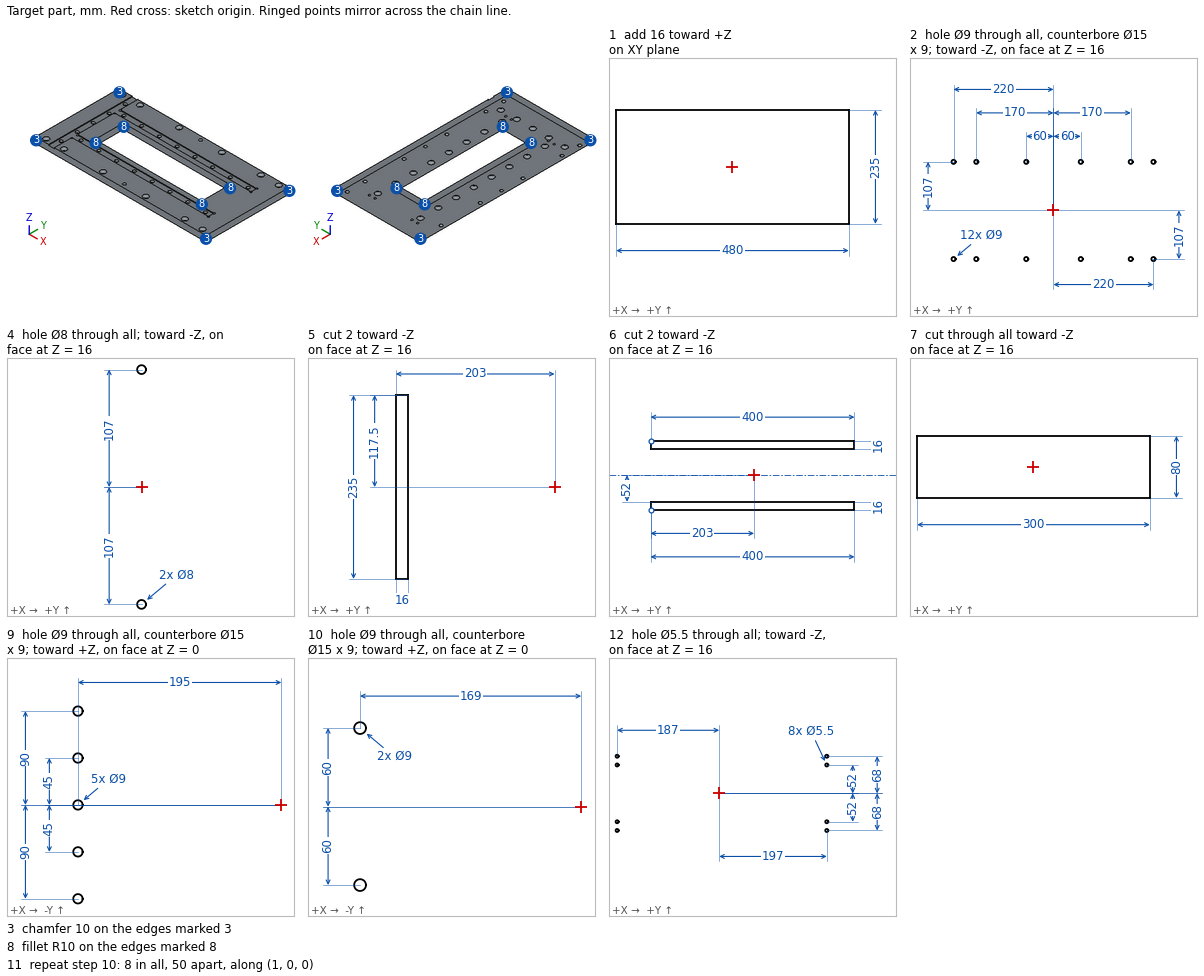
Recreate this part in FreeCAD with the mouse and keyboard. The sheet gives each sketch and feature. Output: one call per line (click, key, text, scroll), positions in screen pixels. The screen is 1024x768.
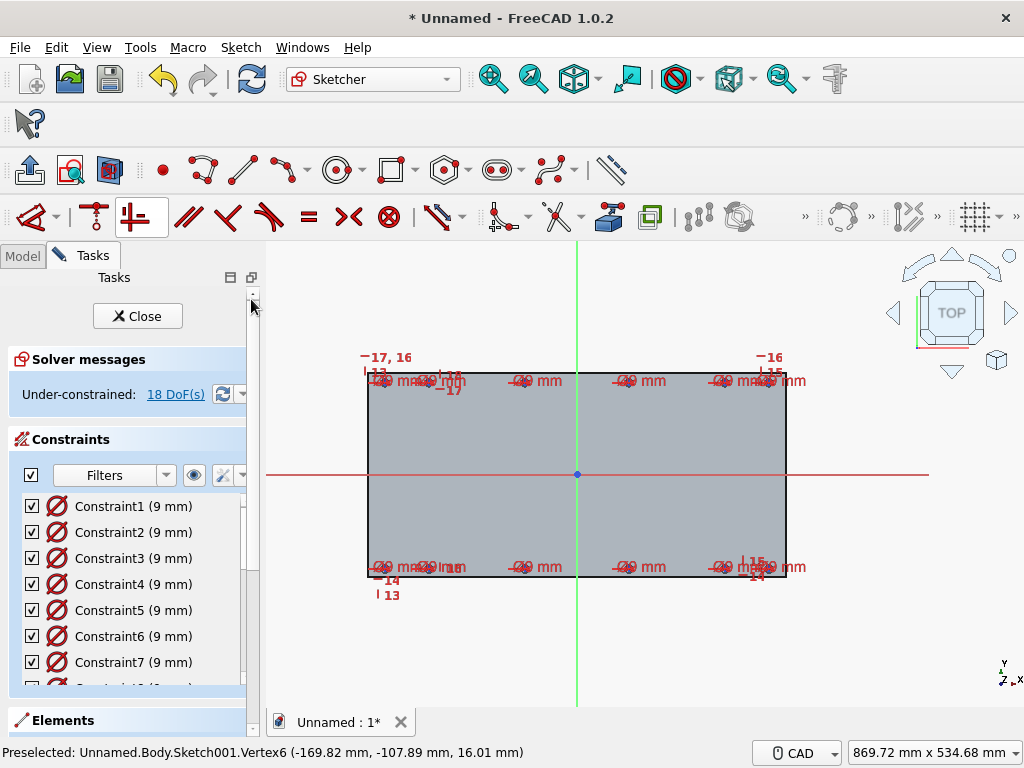
click(385, 569)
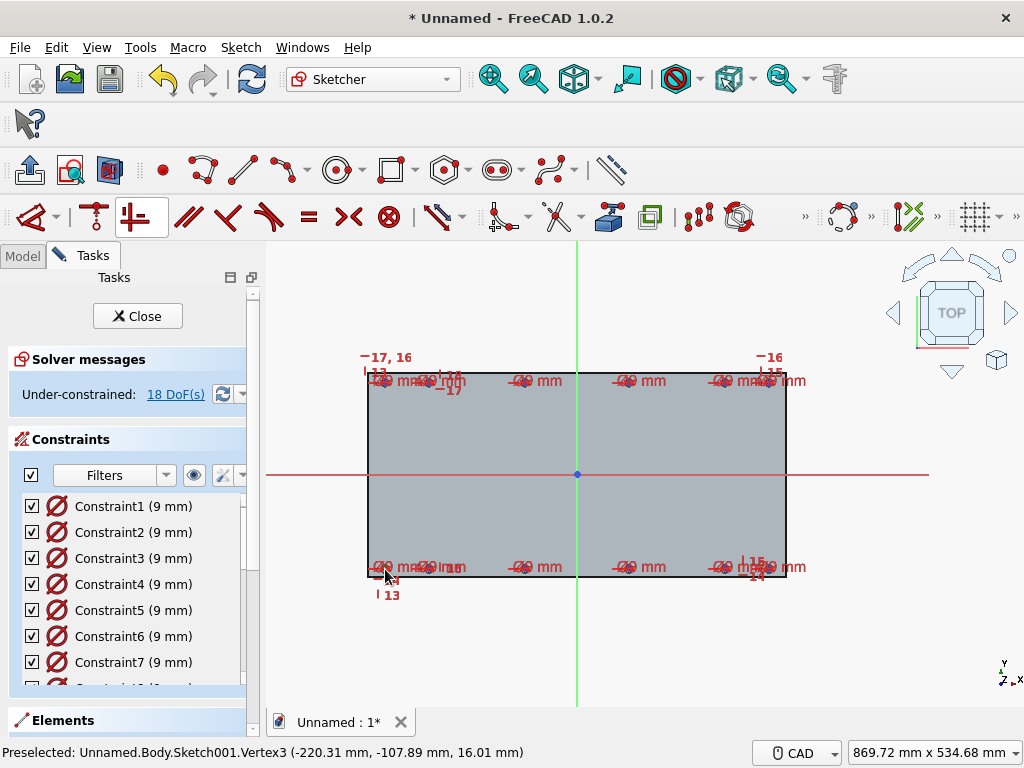
click(429, 569)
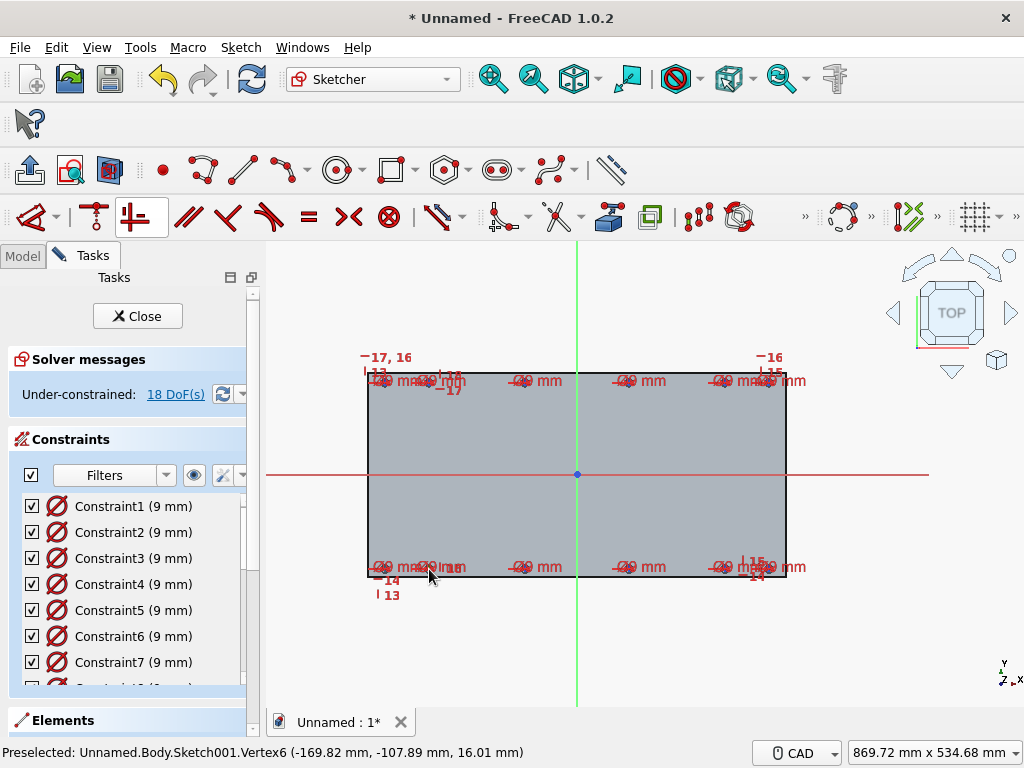
click(162, 218)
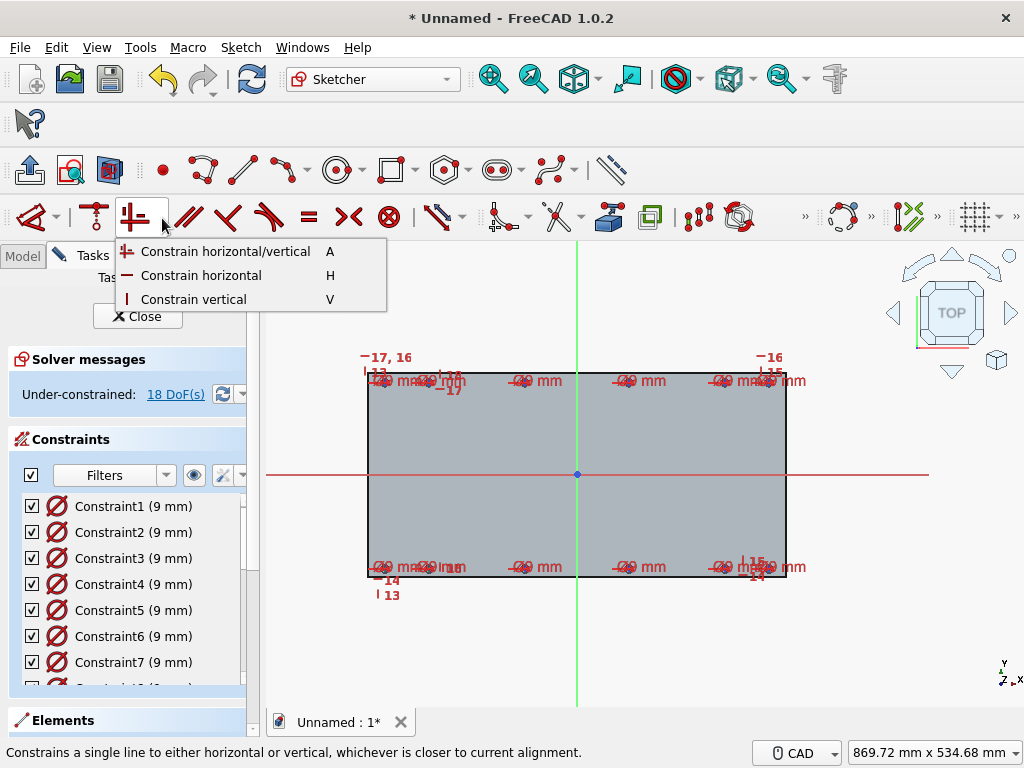
click(251, 275)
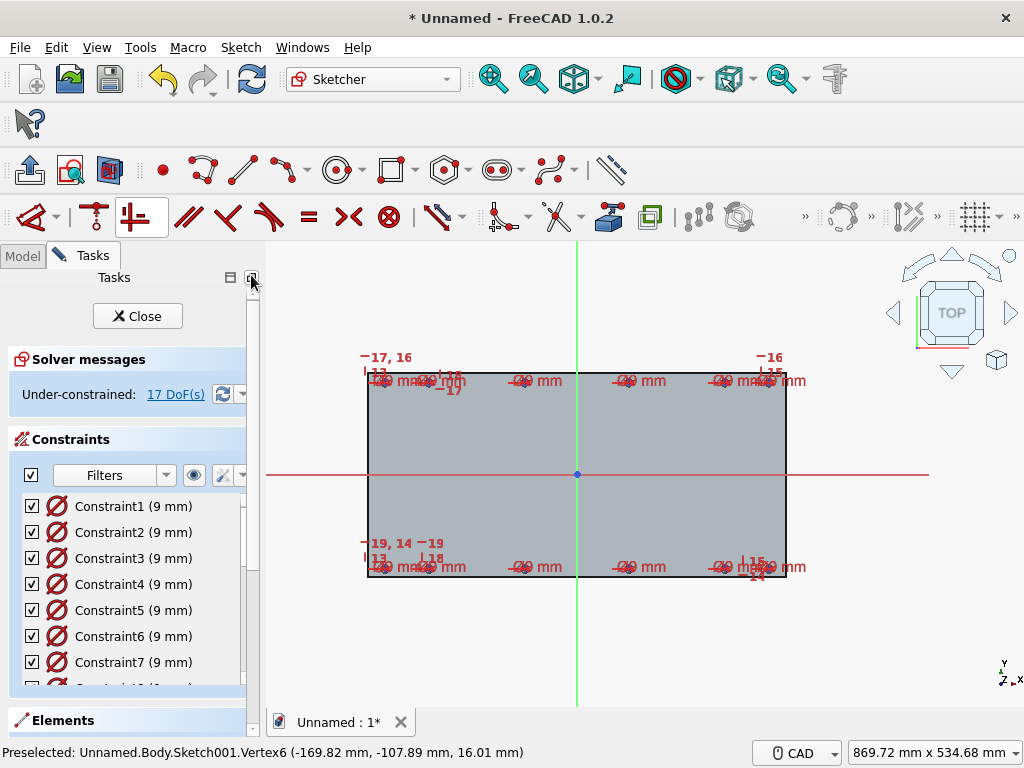
click(429, 383)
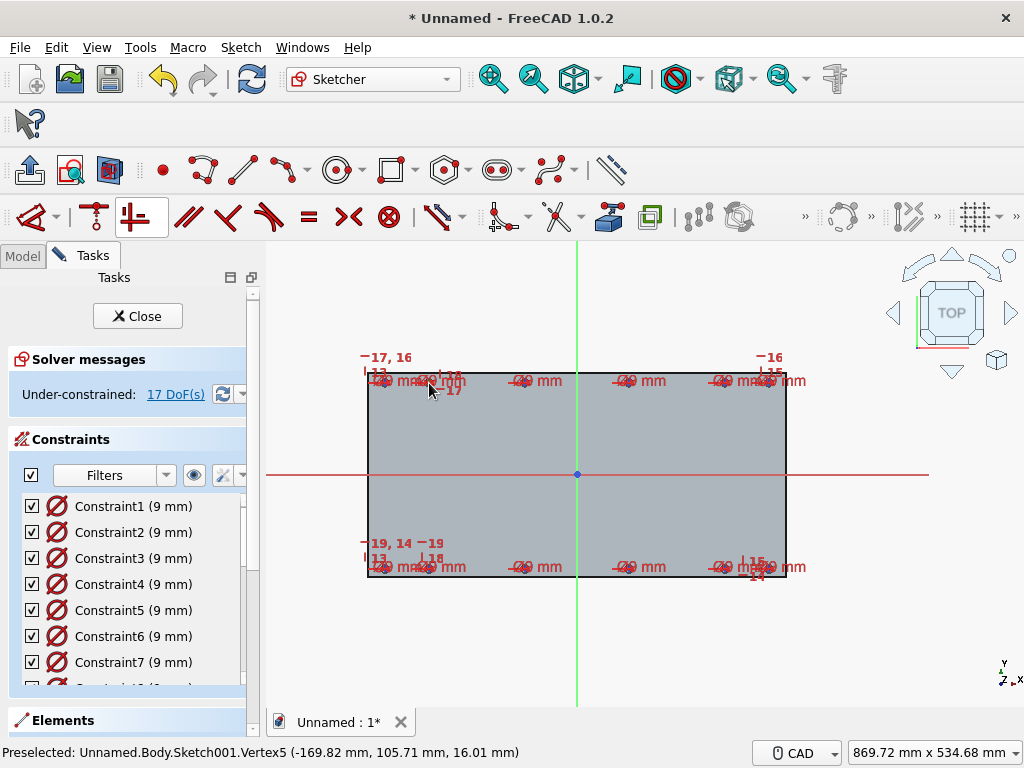
click(525, 383)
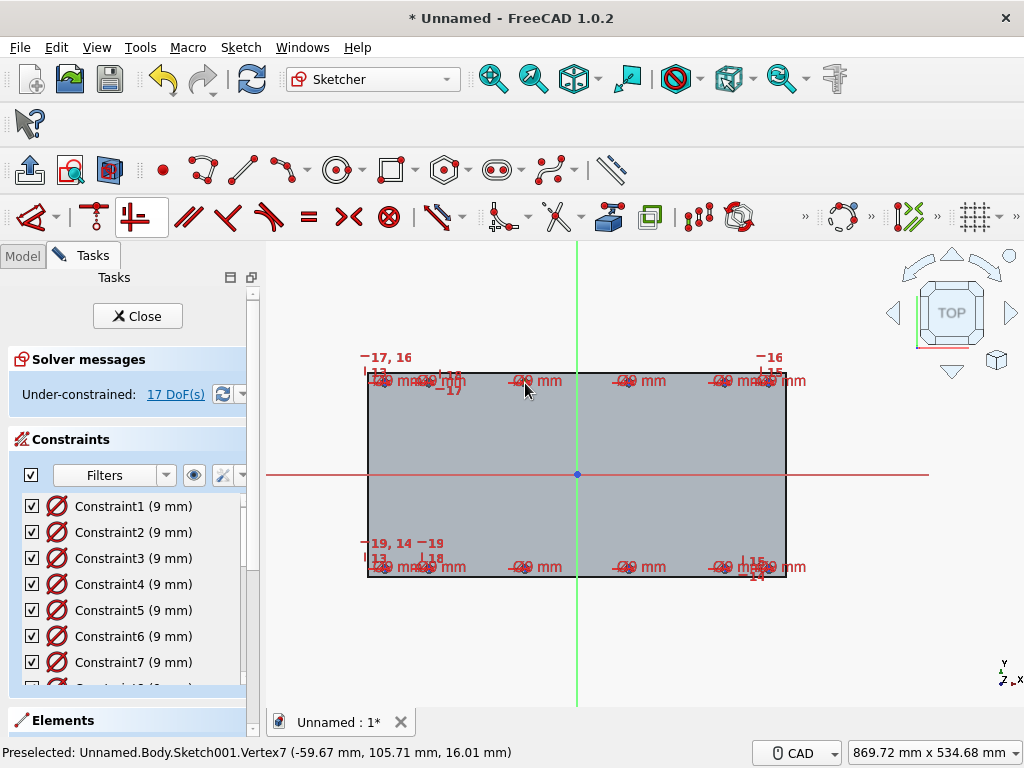
click(162, 218)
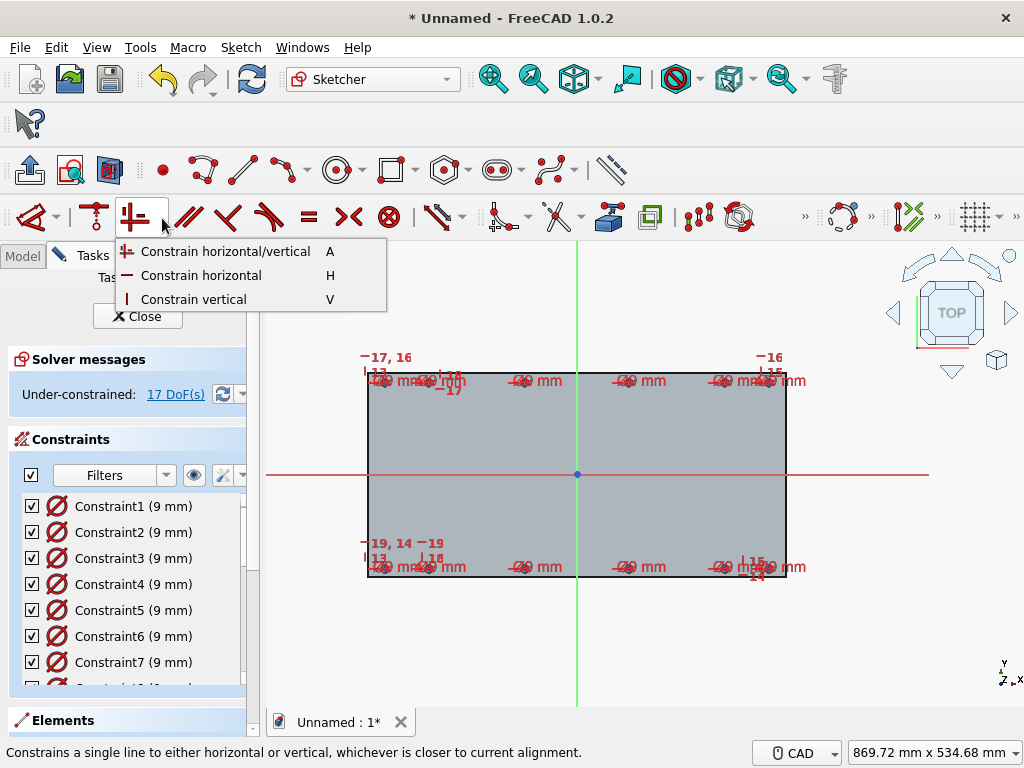
click(251, 275)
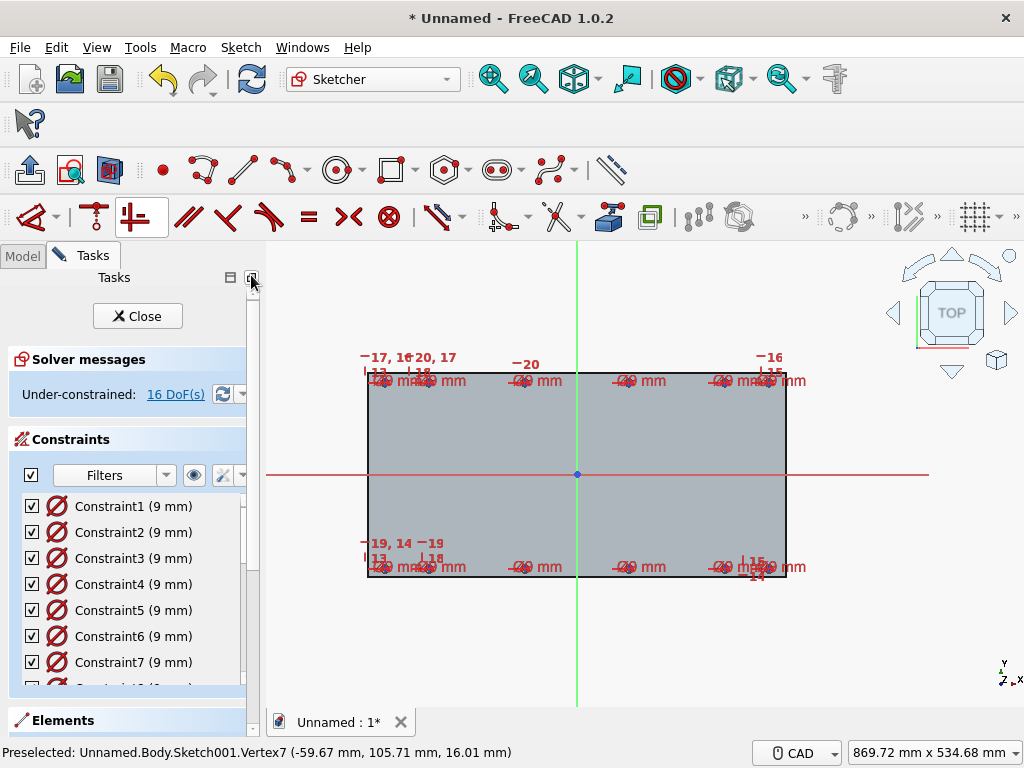
click(525, 383)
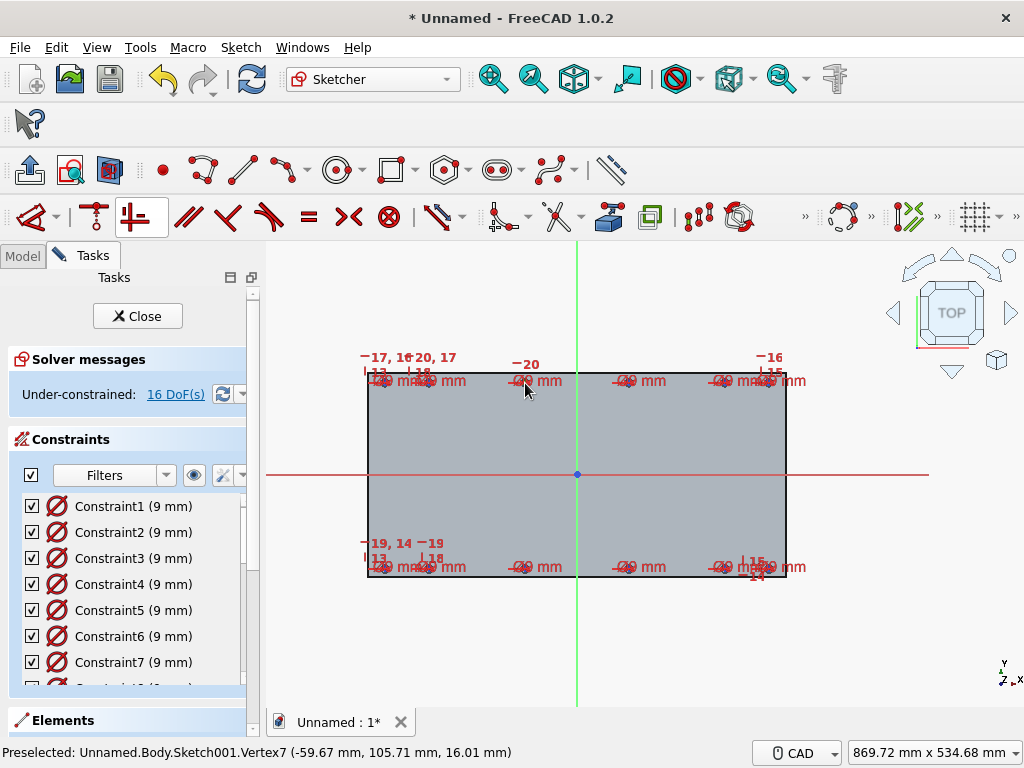
click(525, 569)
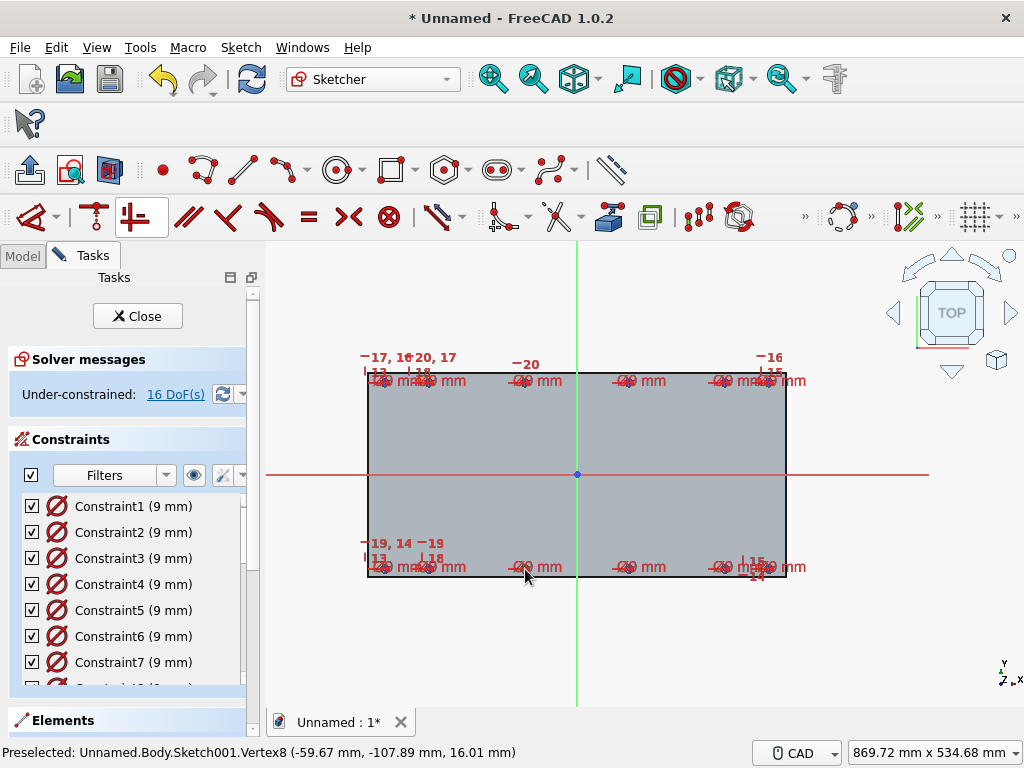
click(162, 218)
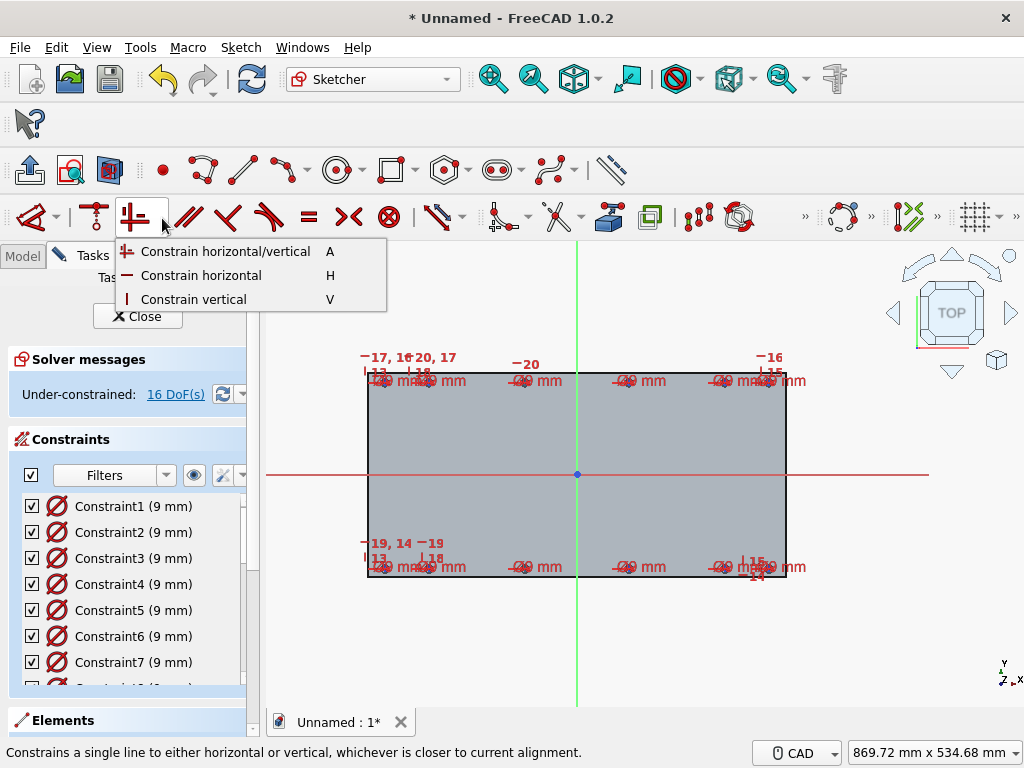
click(251, 299)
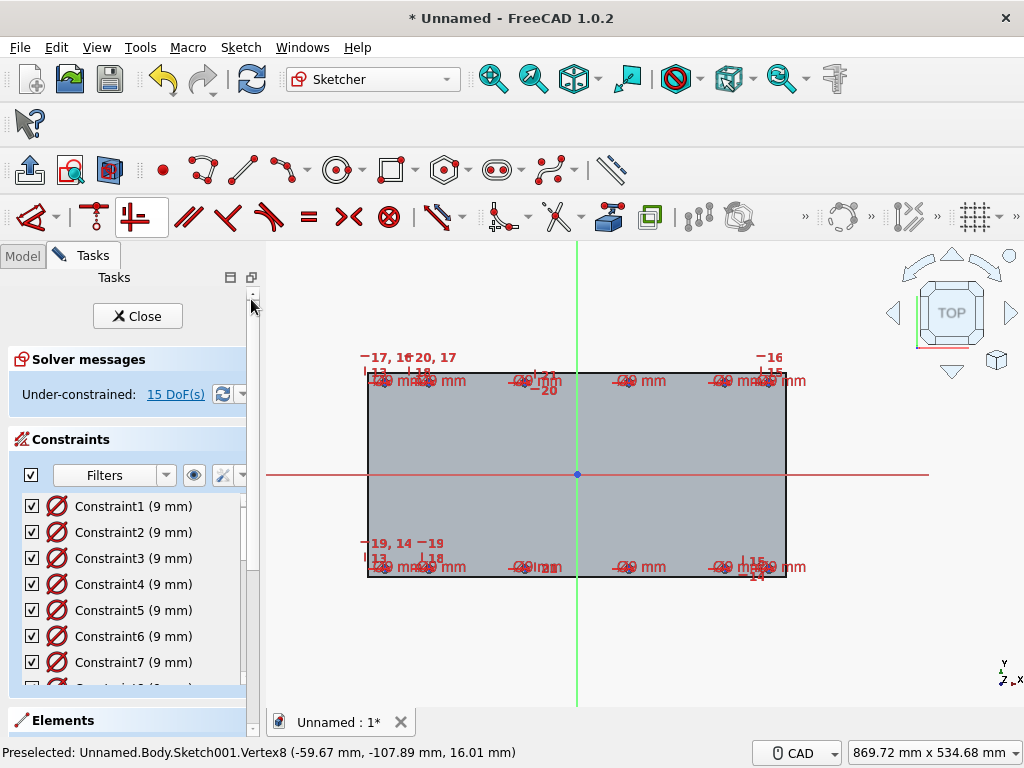
click(429, 569)